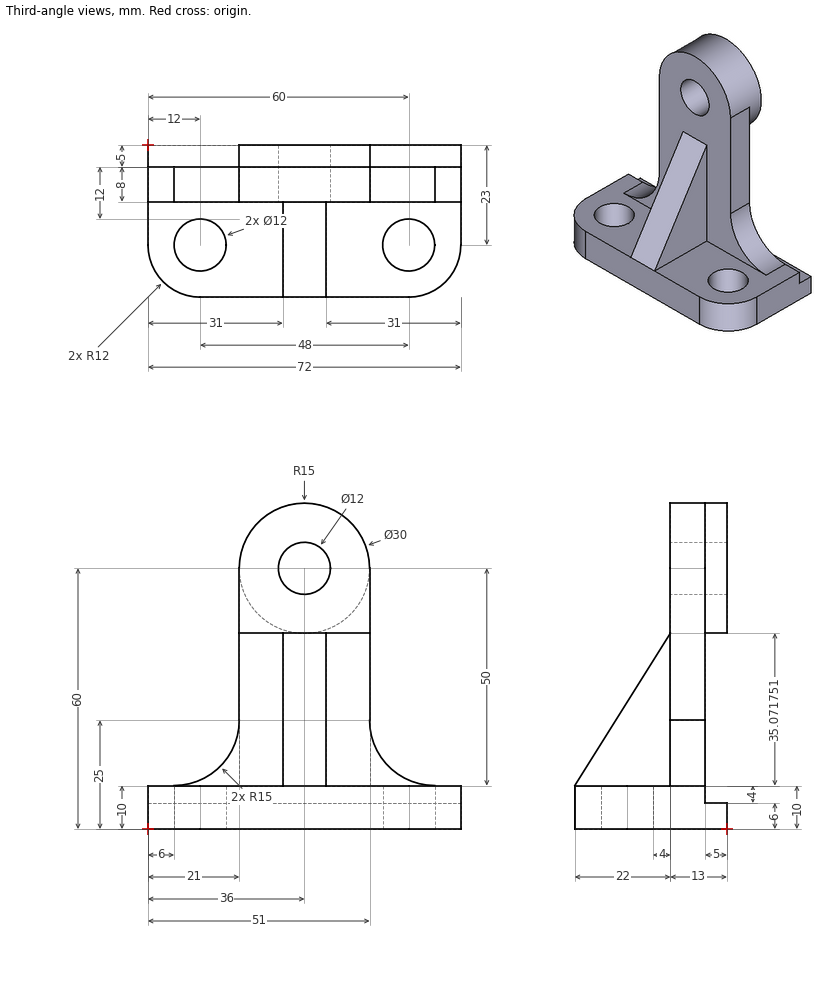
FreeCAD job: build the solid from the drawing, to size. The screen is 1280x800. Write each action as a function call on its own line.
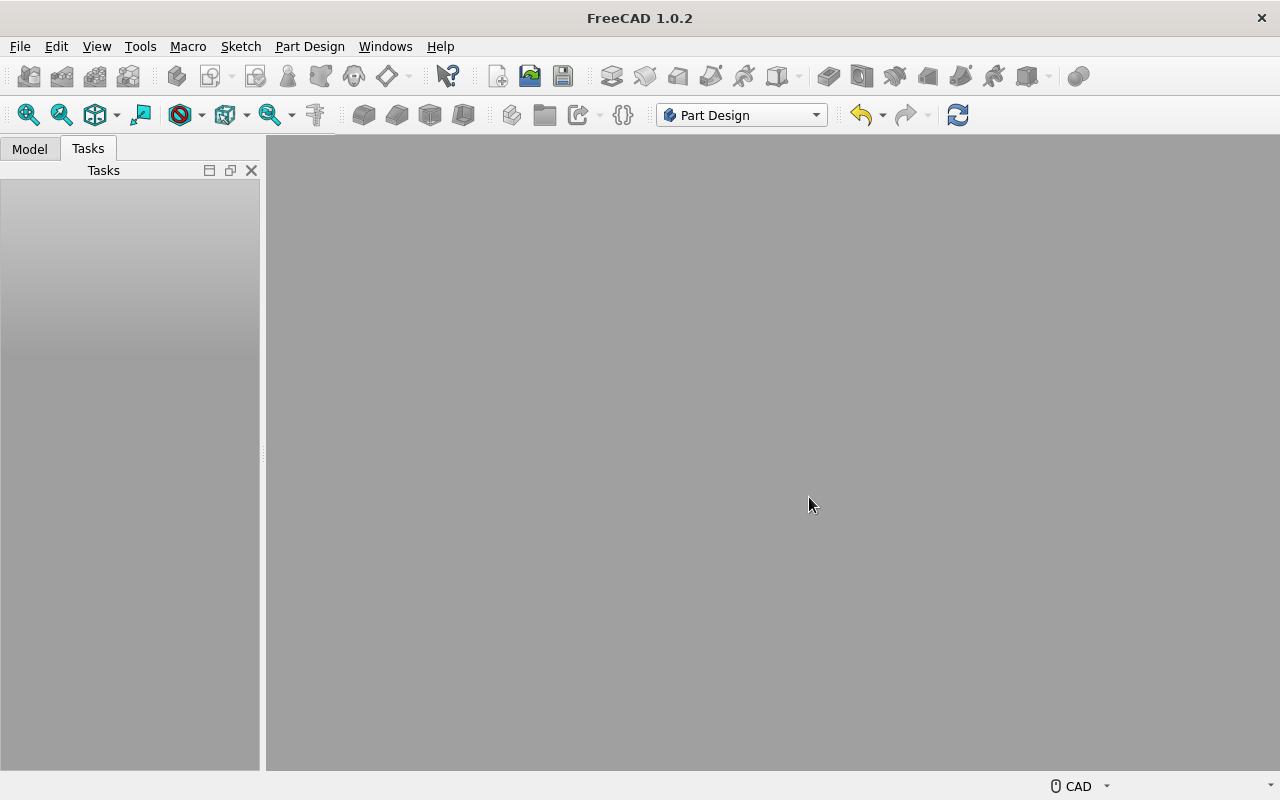
click(497, 76)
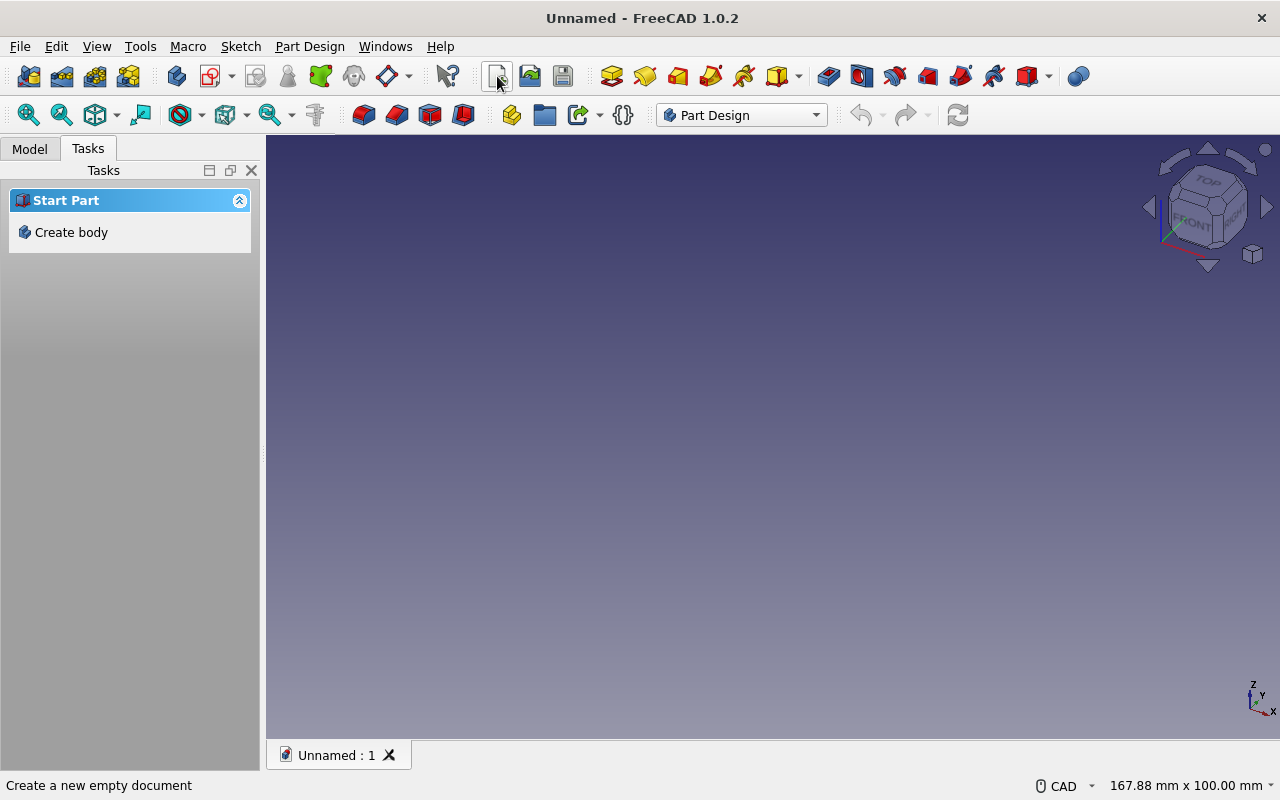
click(210, 76)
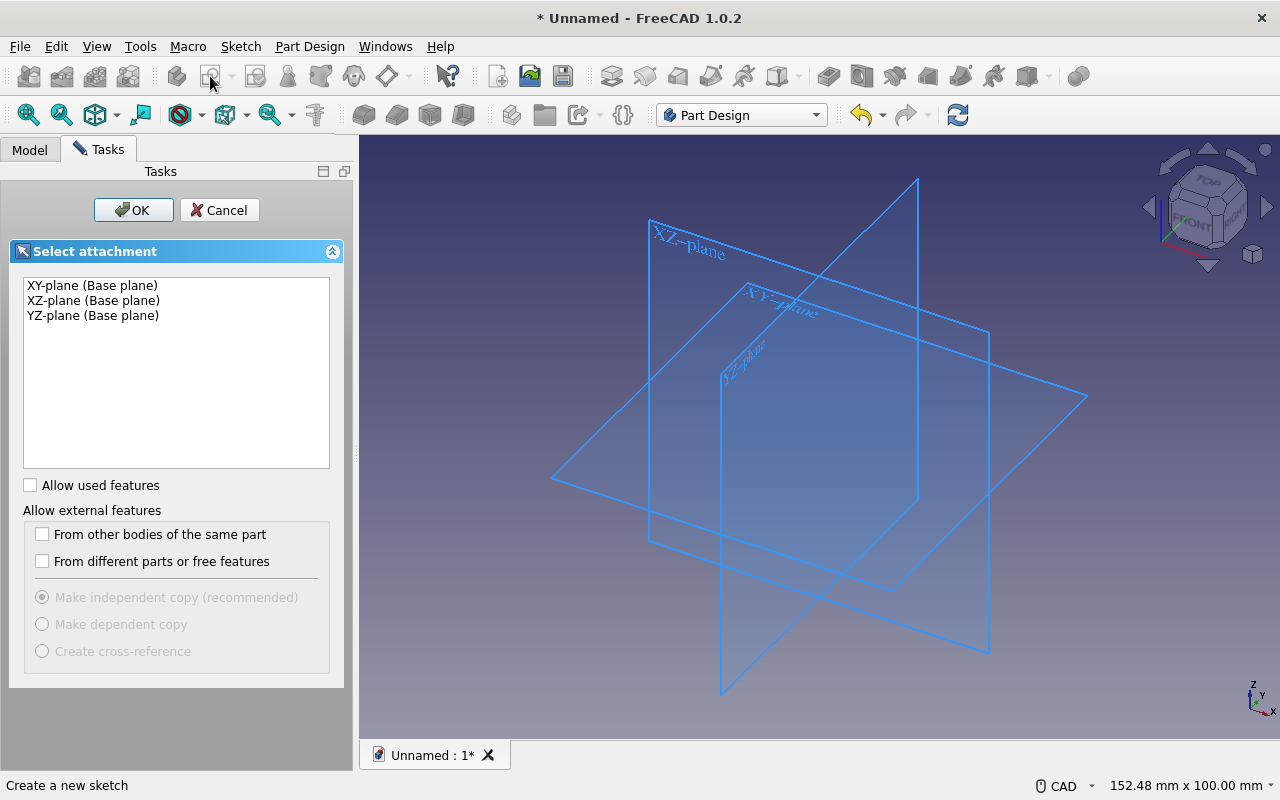
click(84, 286)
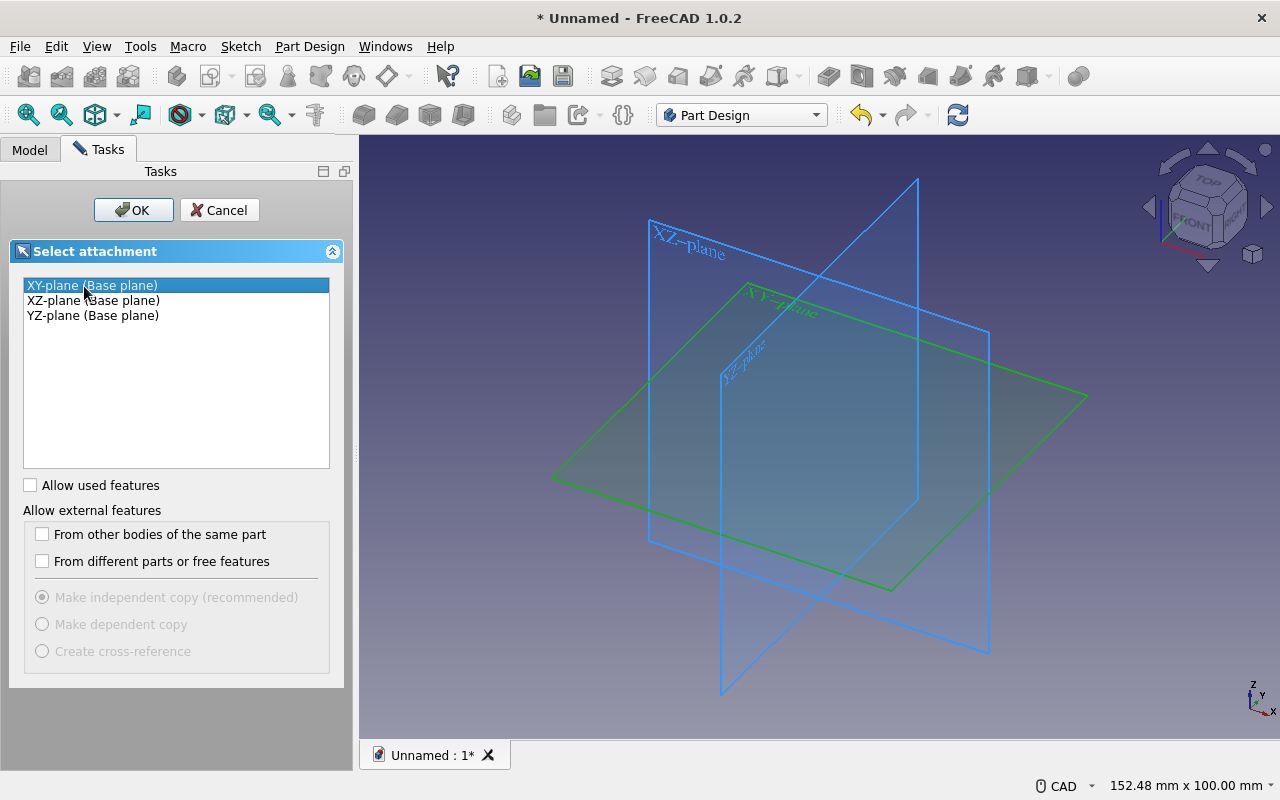
click(134, 210)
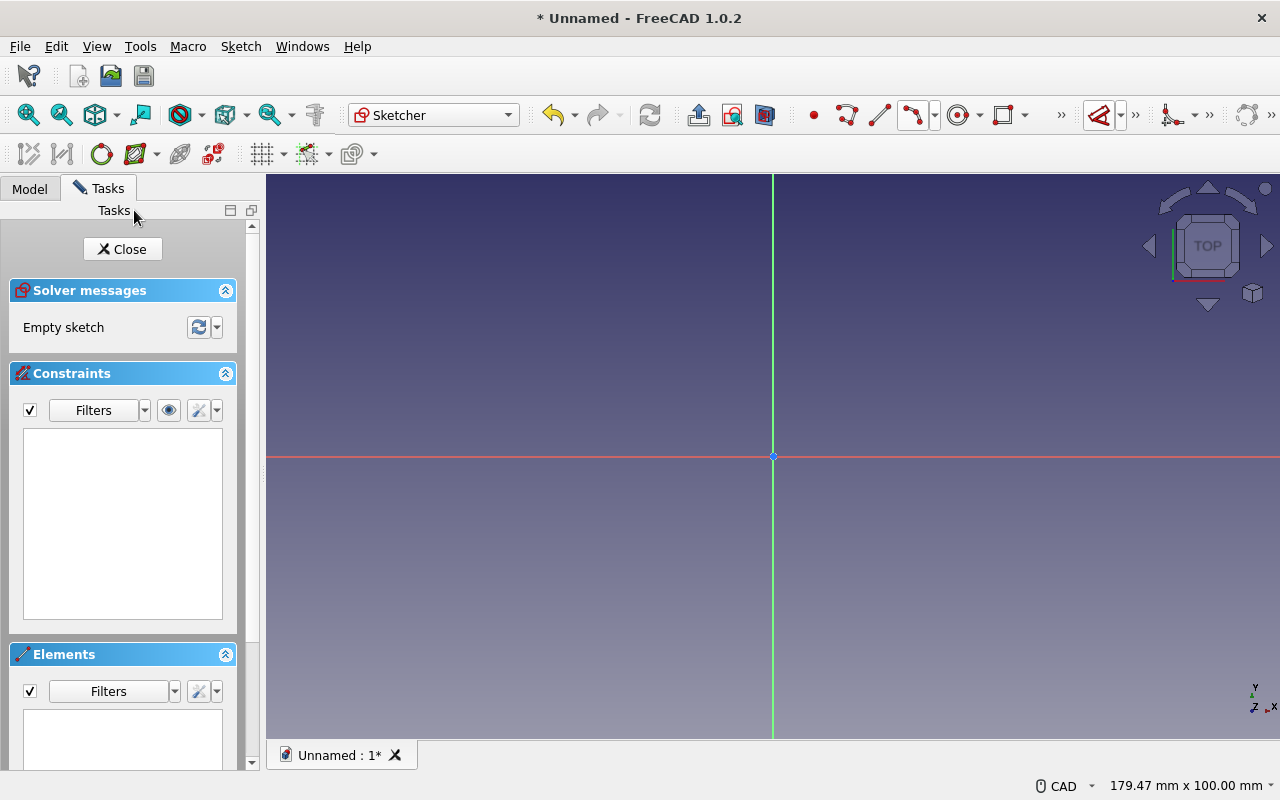
scroll(294, 202, down, 1)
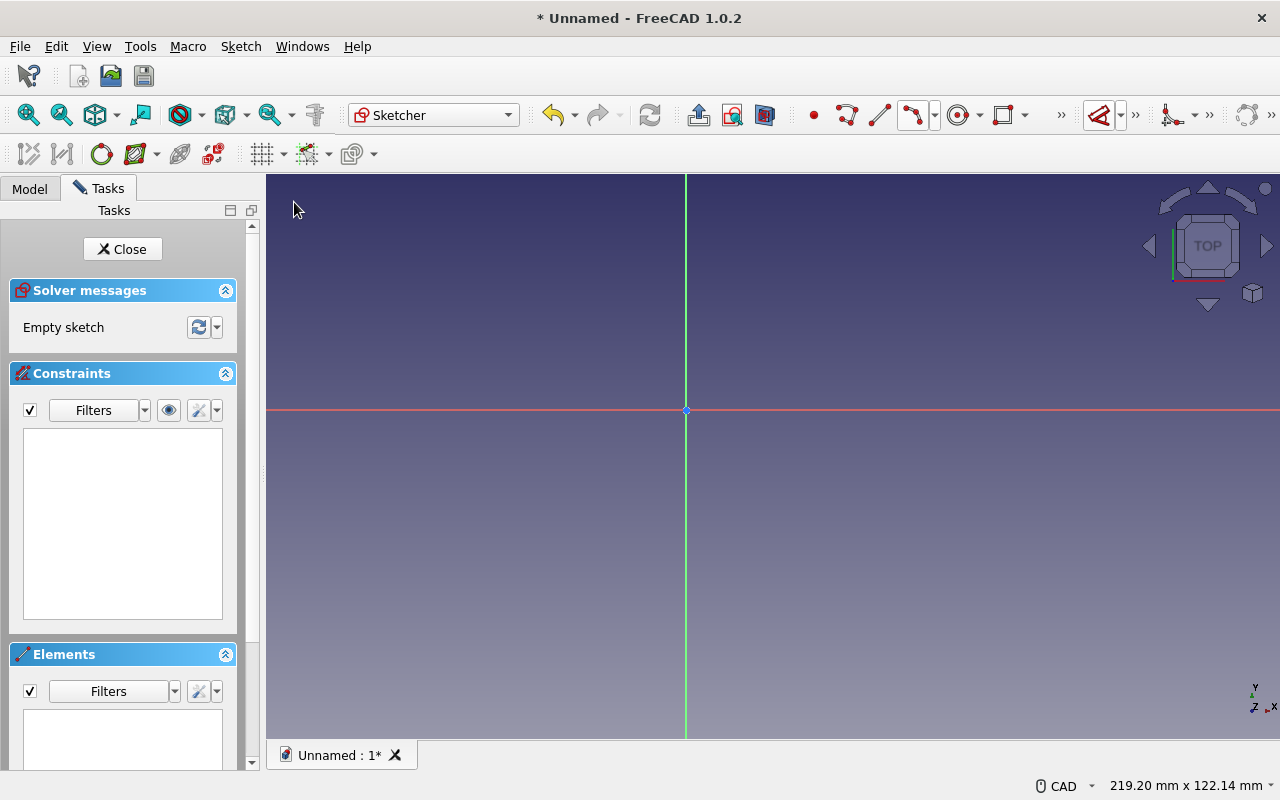
scroll(1033, 534, up, 3)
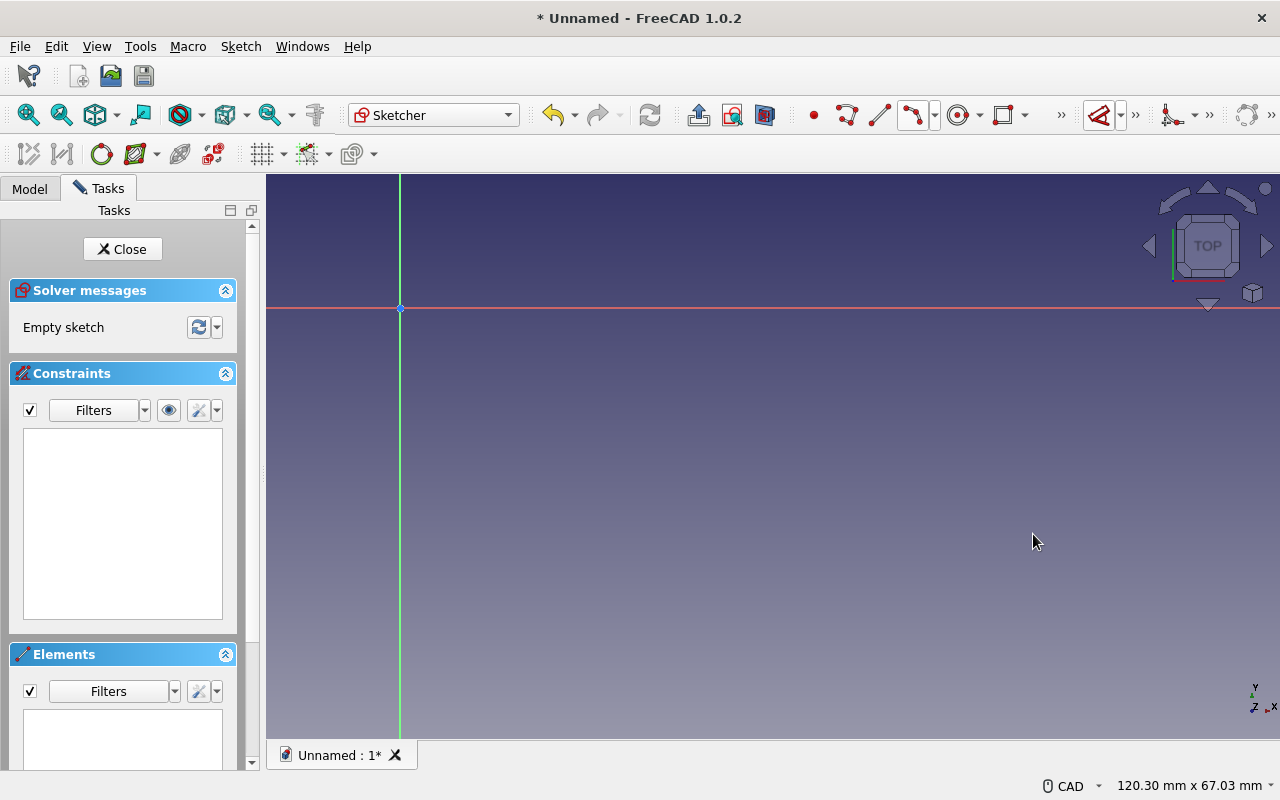
click(880, 116)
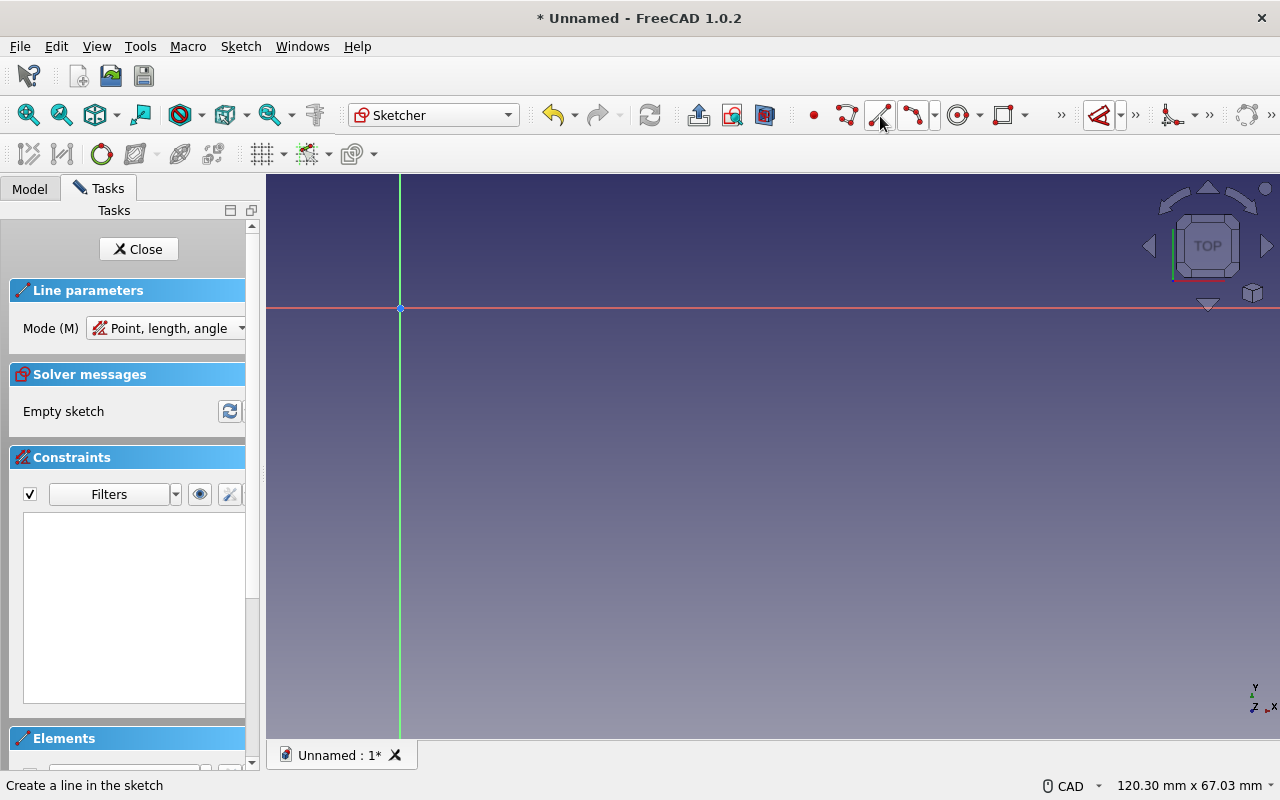
click(502, 603)
click(906, 603)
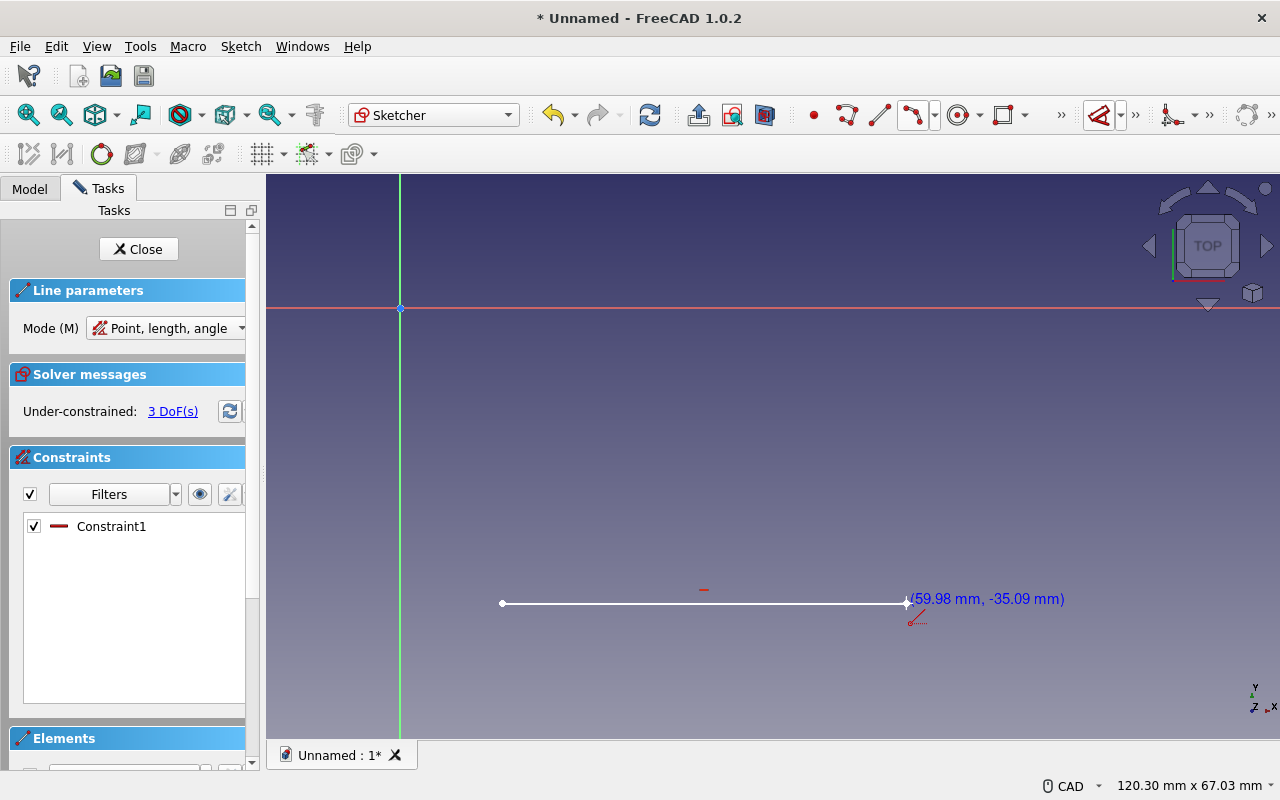
click(847, 116)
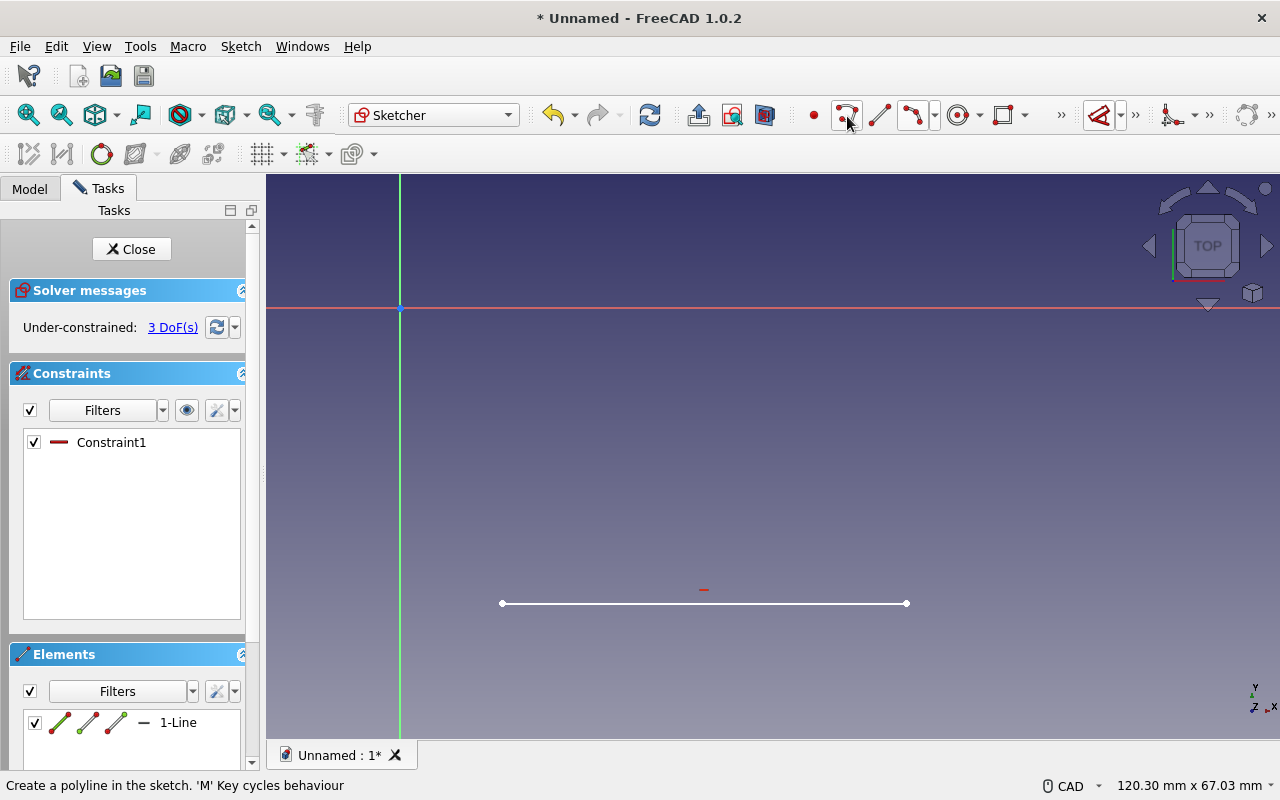
click(1007, 502)
click(1007, 308)
click(400, 308)
click(409, 502)
right_click(409, 502)